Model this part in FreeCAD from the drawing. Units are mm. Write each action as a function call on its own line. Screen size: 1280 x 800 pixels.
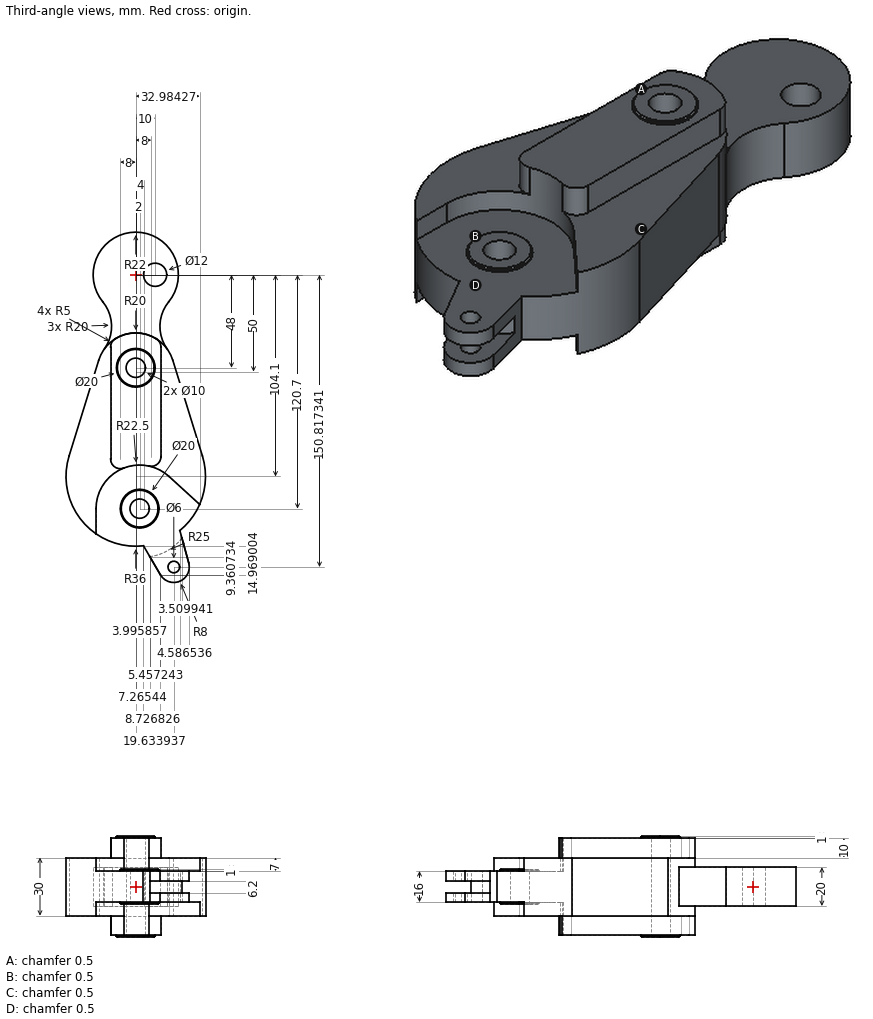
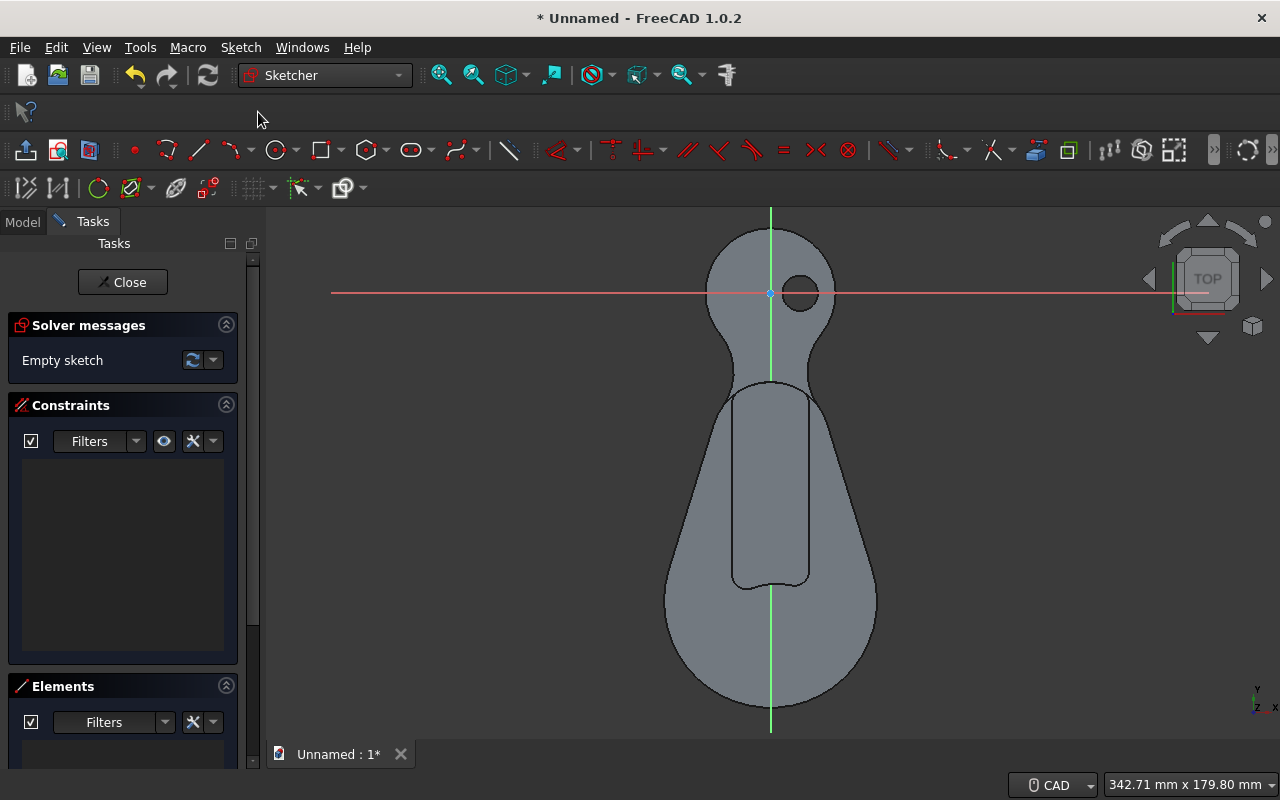
click(90, 150)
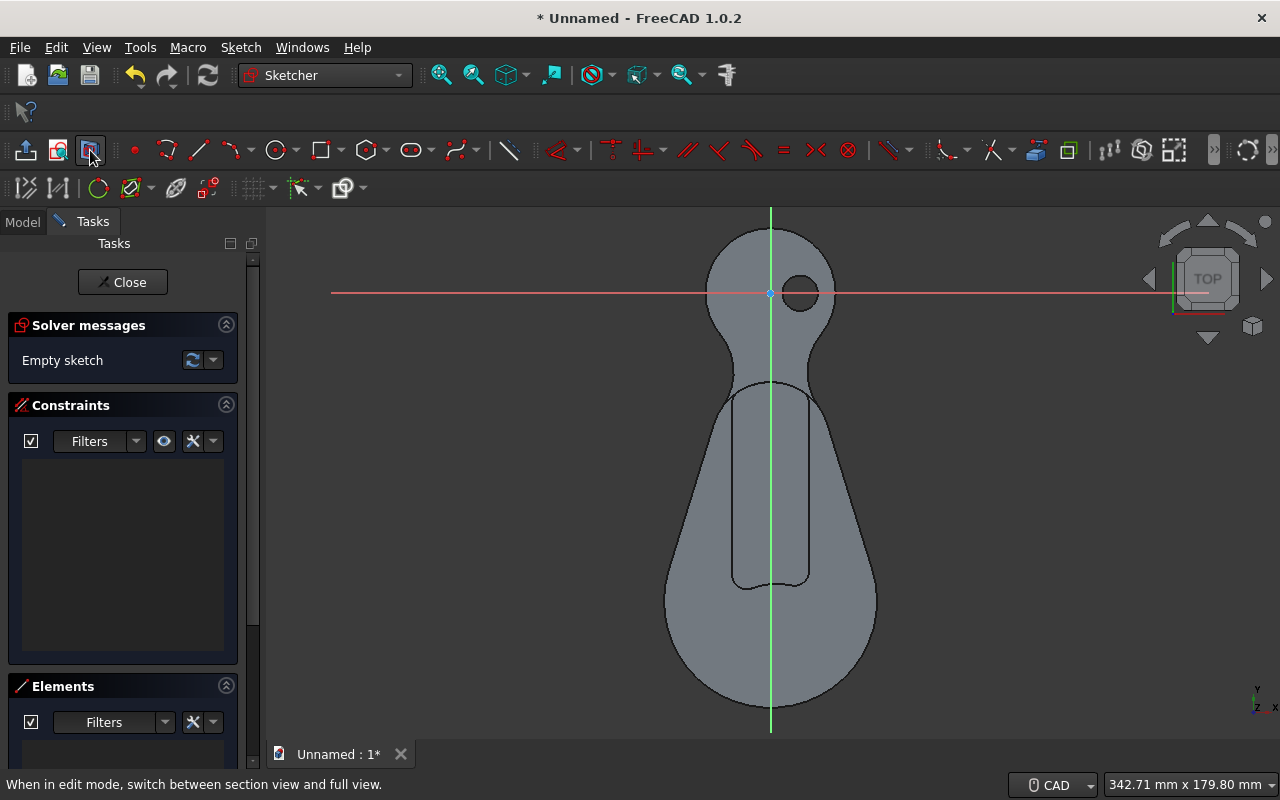
scroll(704, 473, down, 5)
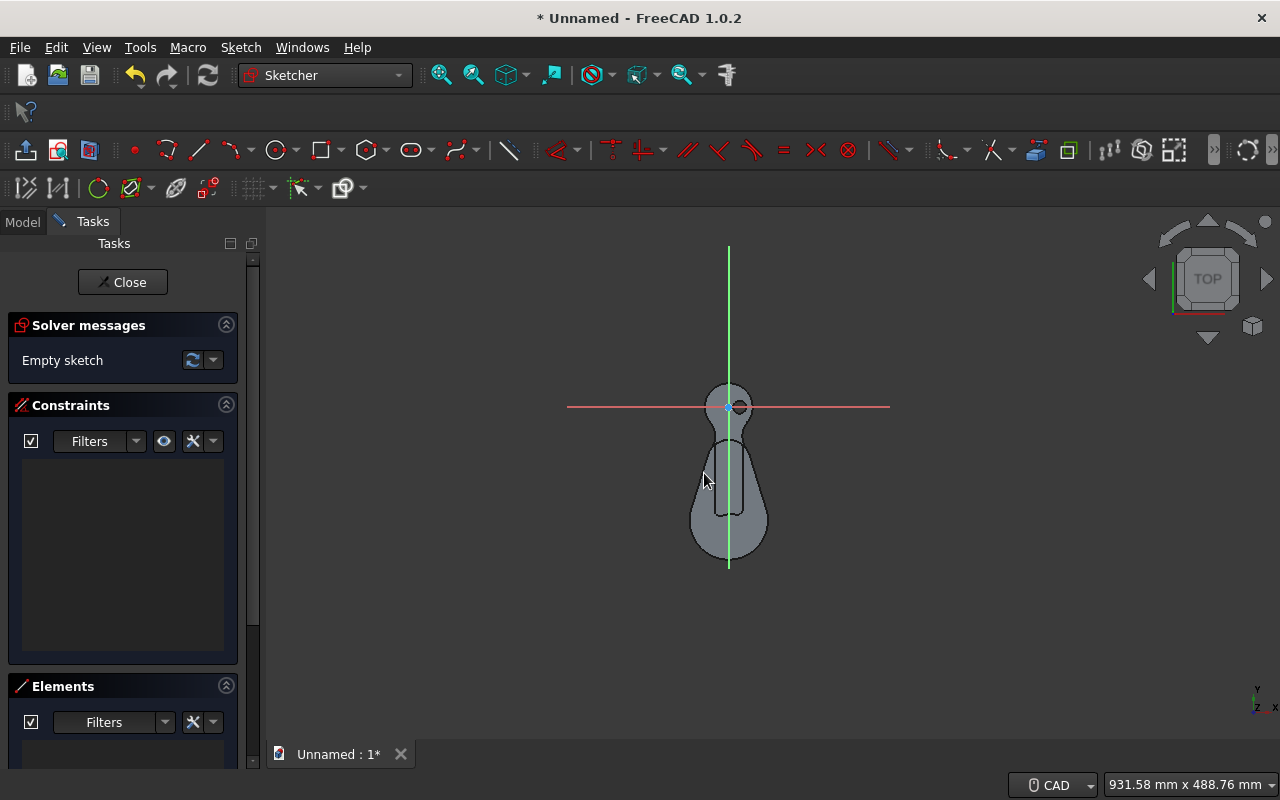
scroll(740, 547, up, 10)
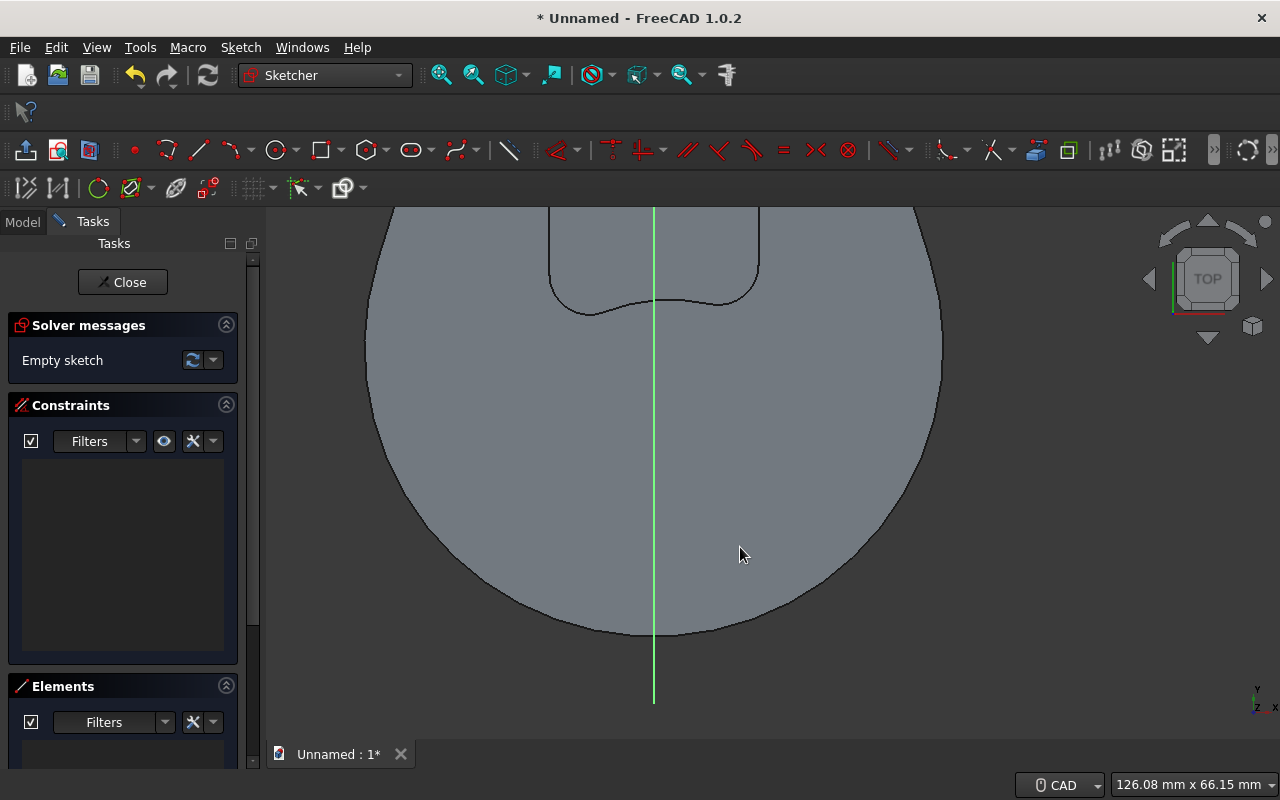
click(200, 150)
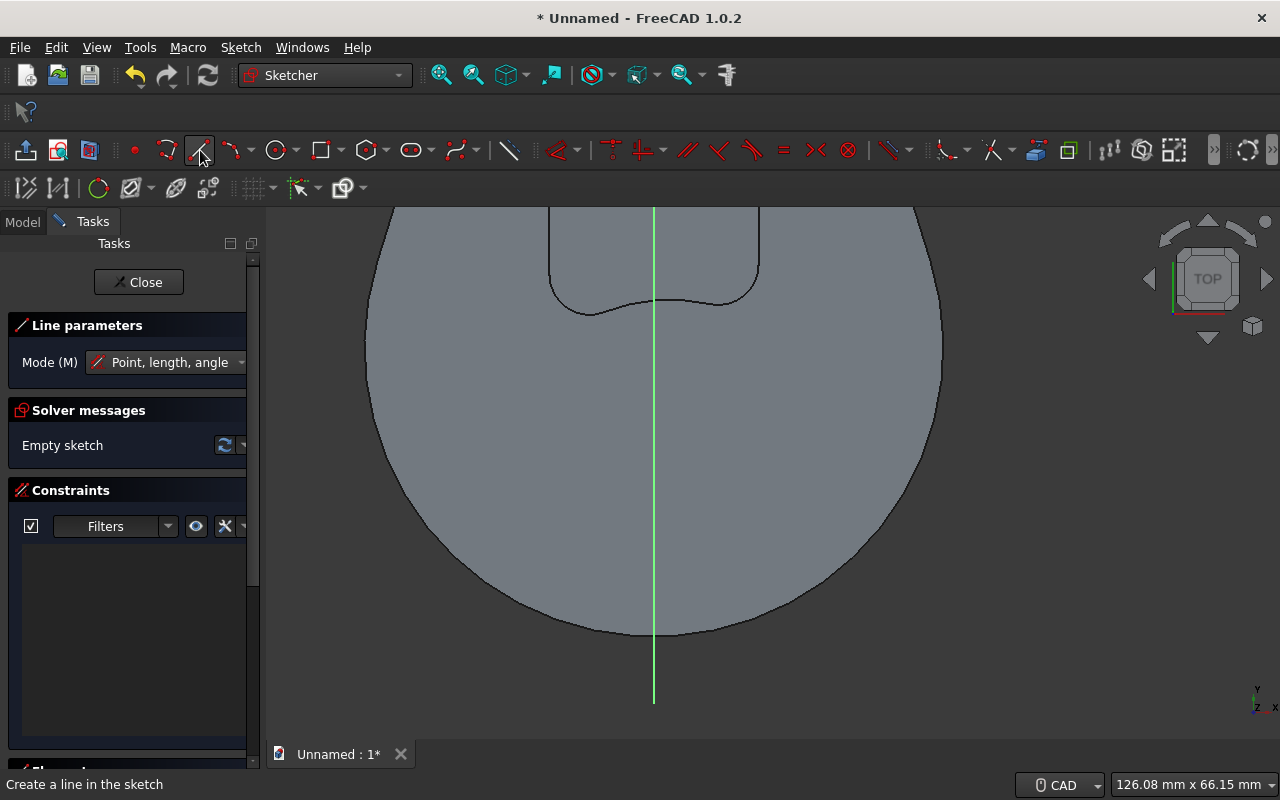
click(489, 481)
click(489, 585)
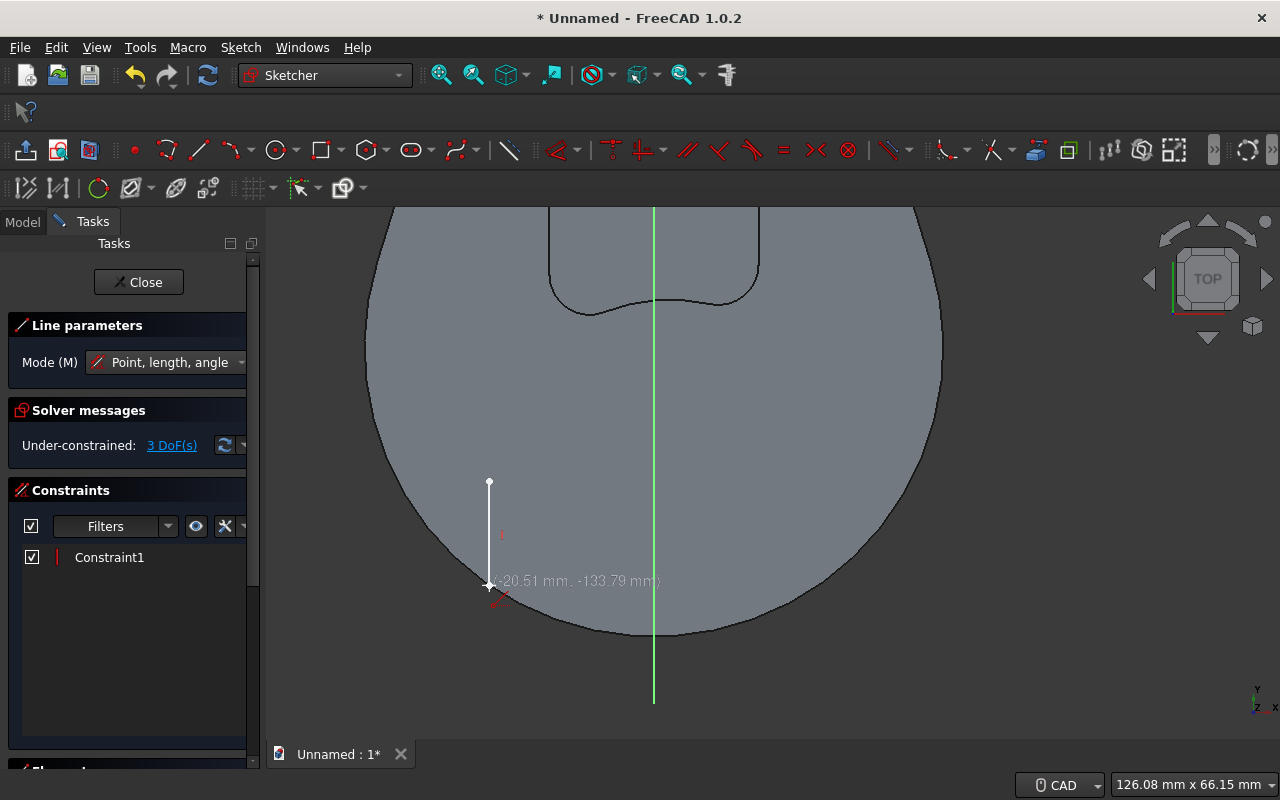
click(919, 463)
click(792, 347)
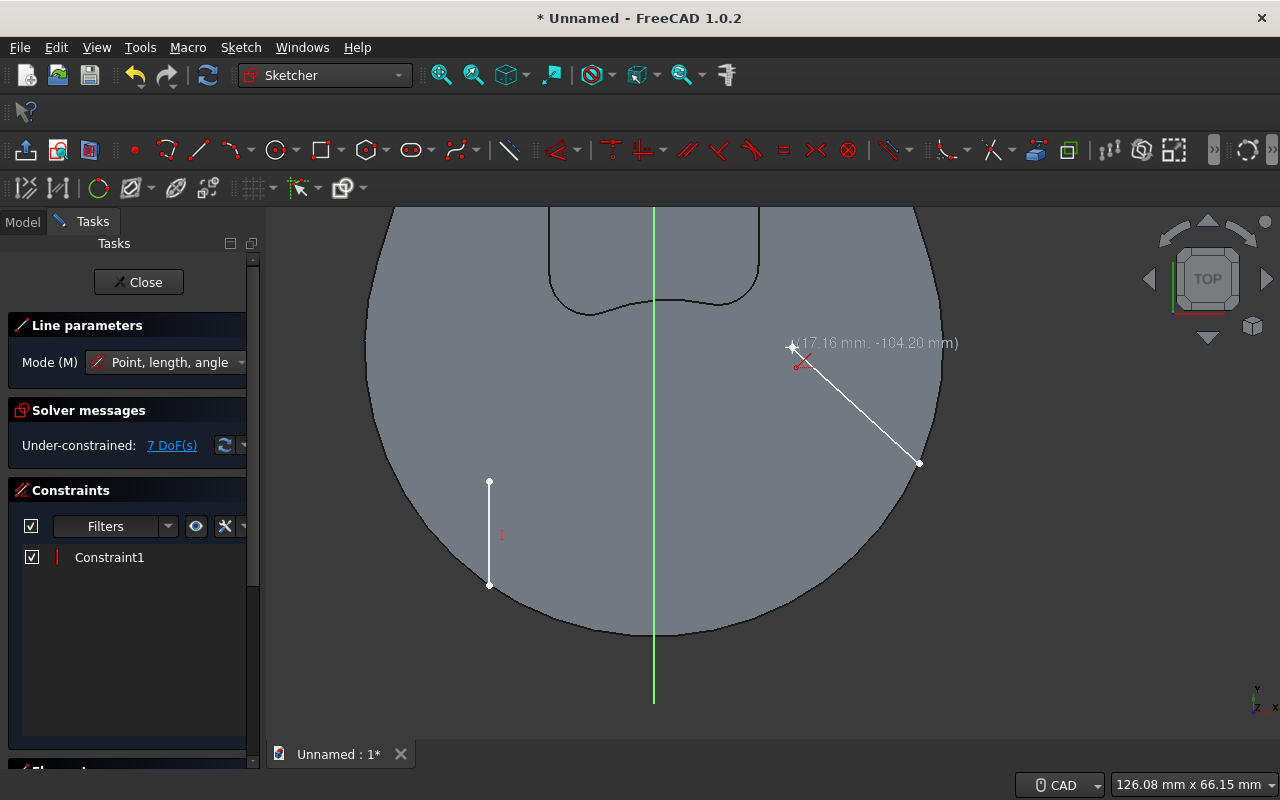
click(232, 150)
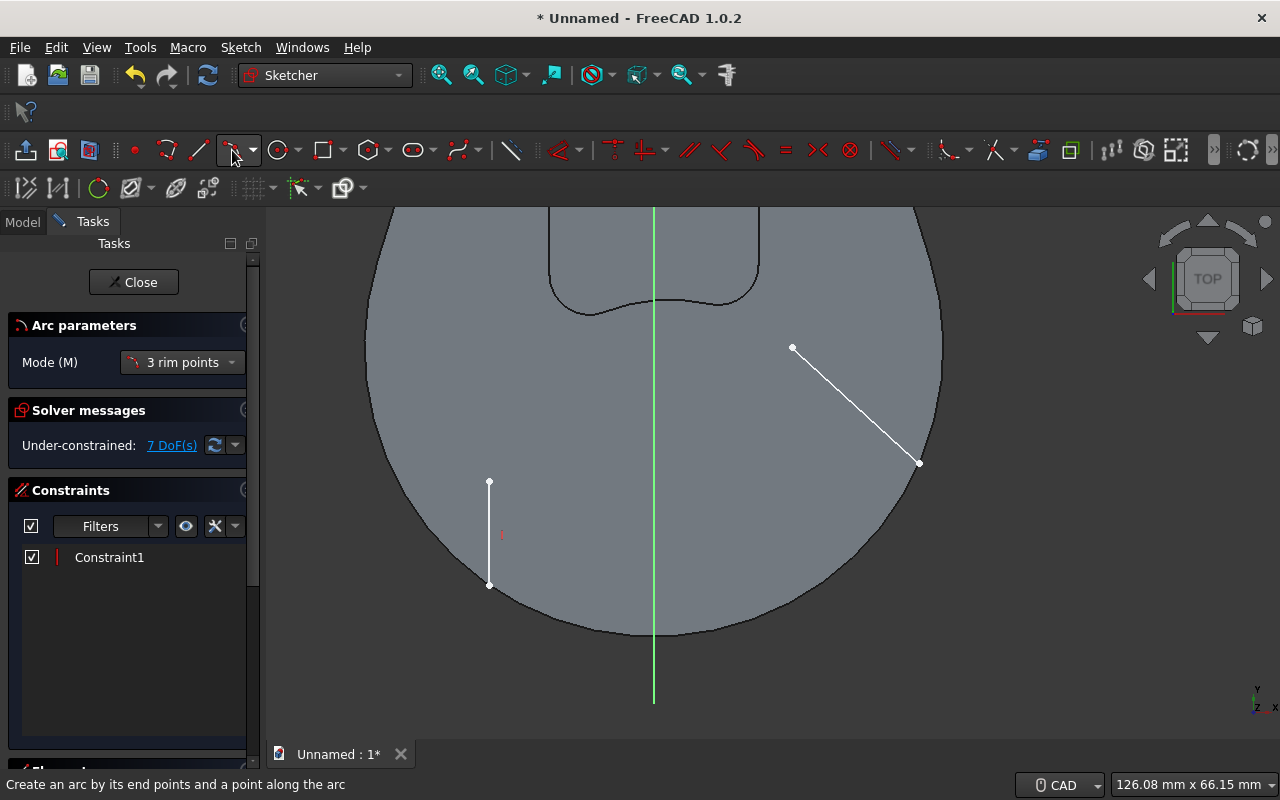
click(489, 586)
click(919, 464)
click(733, 626)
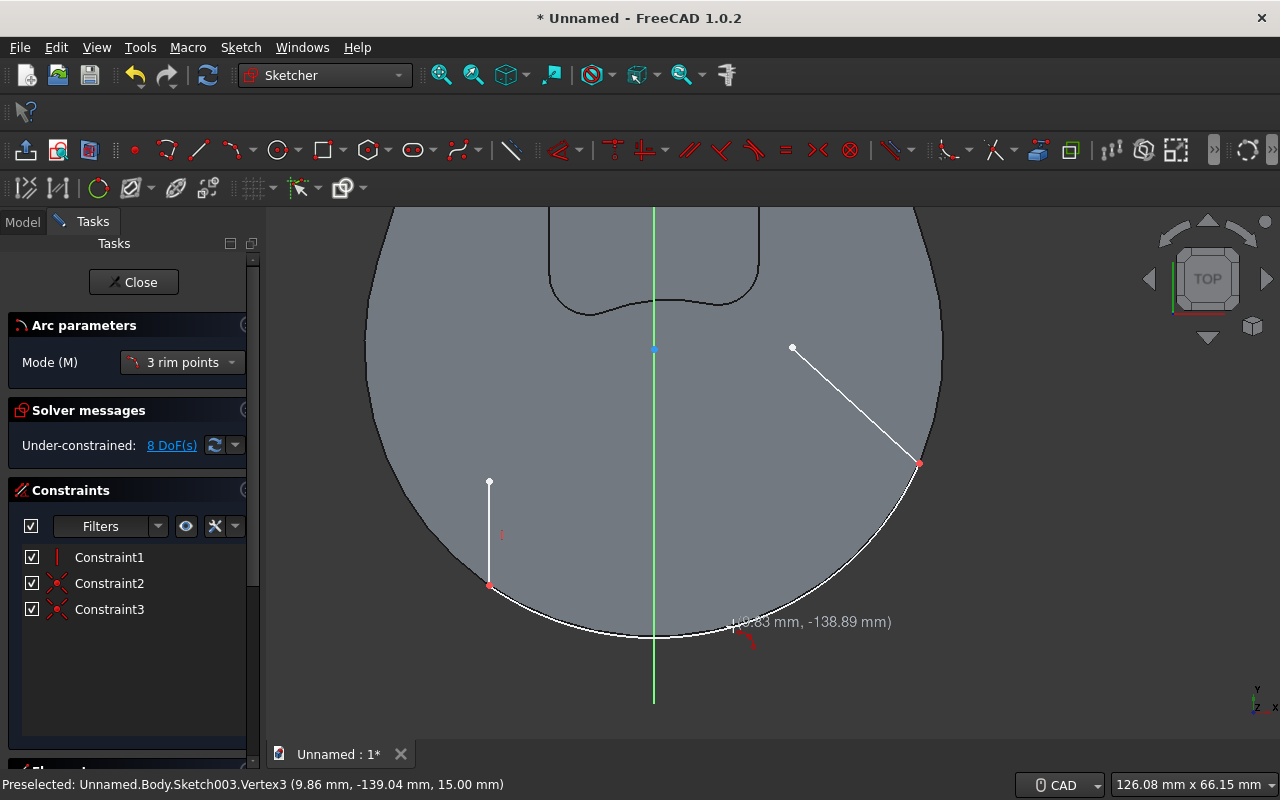
click(792, 348)
click(489, 482)
click(597, 315)
key(Escape)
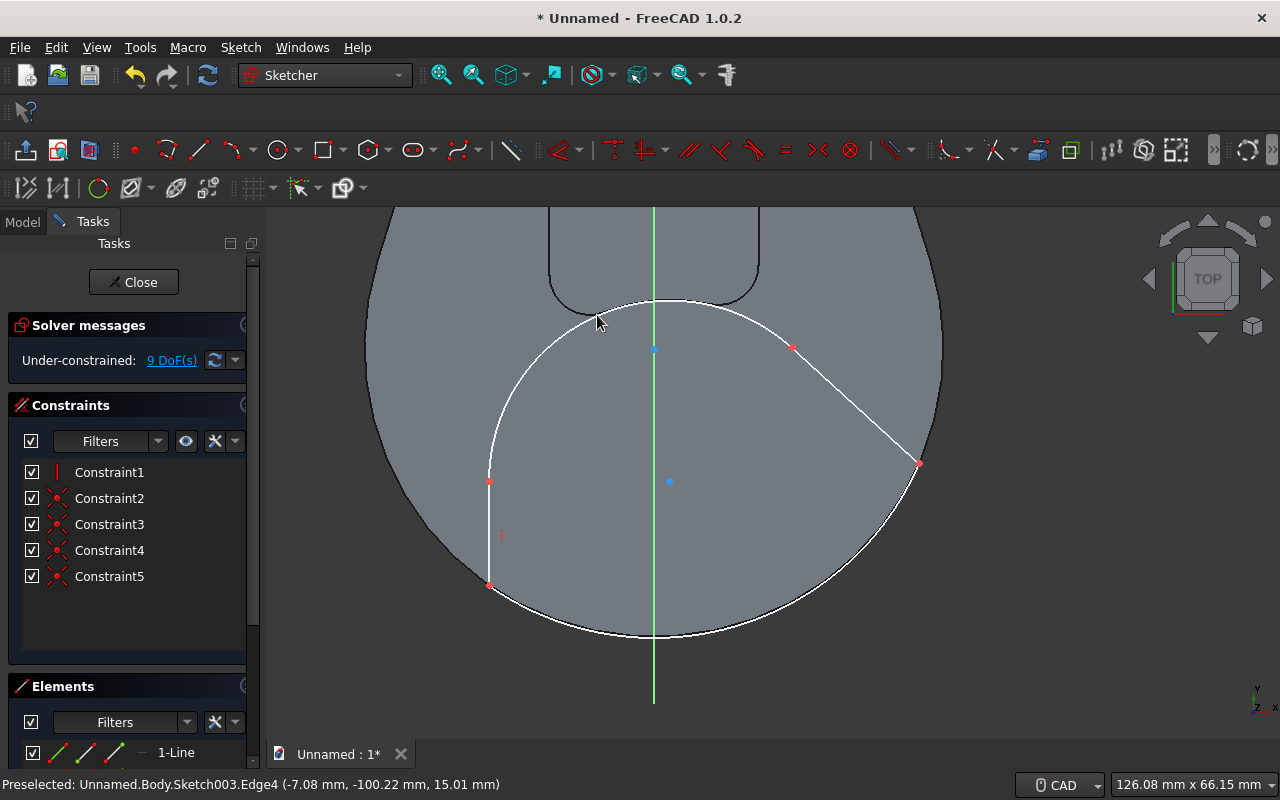
click(489, 513)